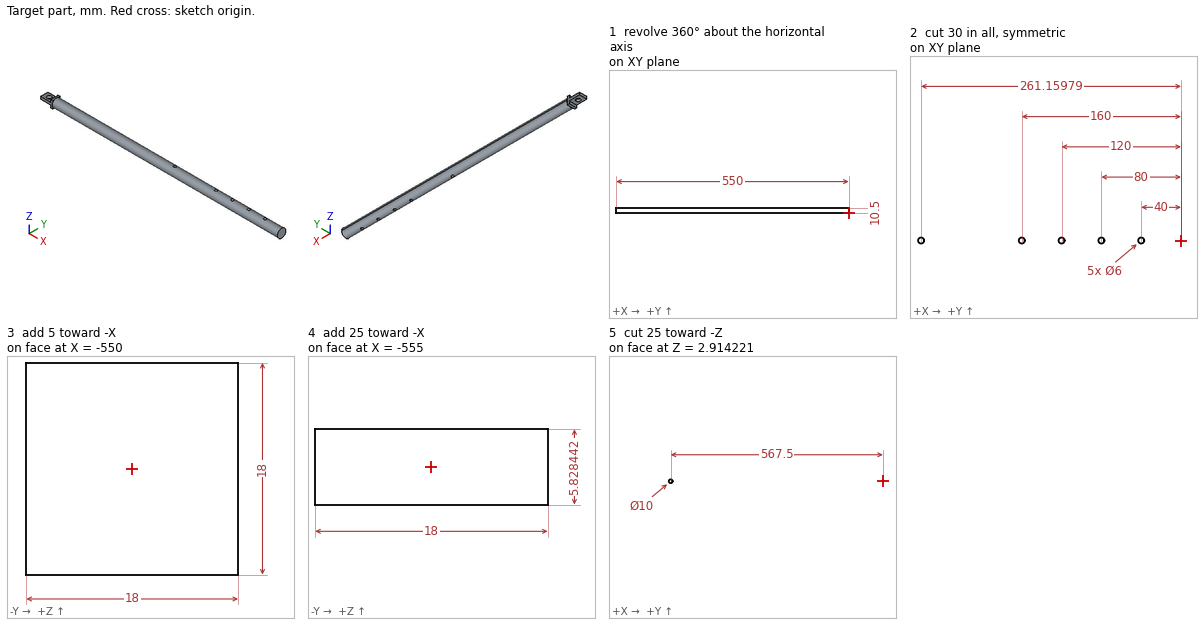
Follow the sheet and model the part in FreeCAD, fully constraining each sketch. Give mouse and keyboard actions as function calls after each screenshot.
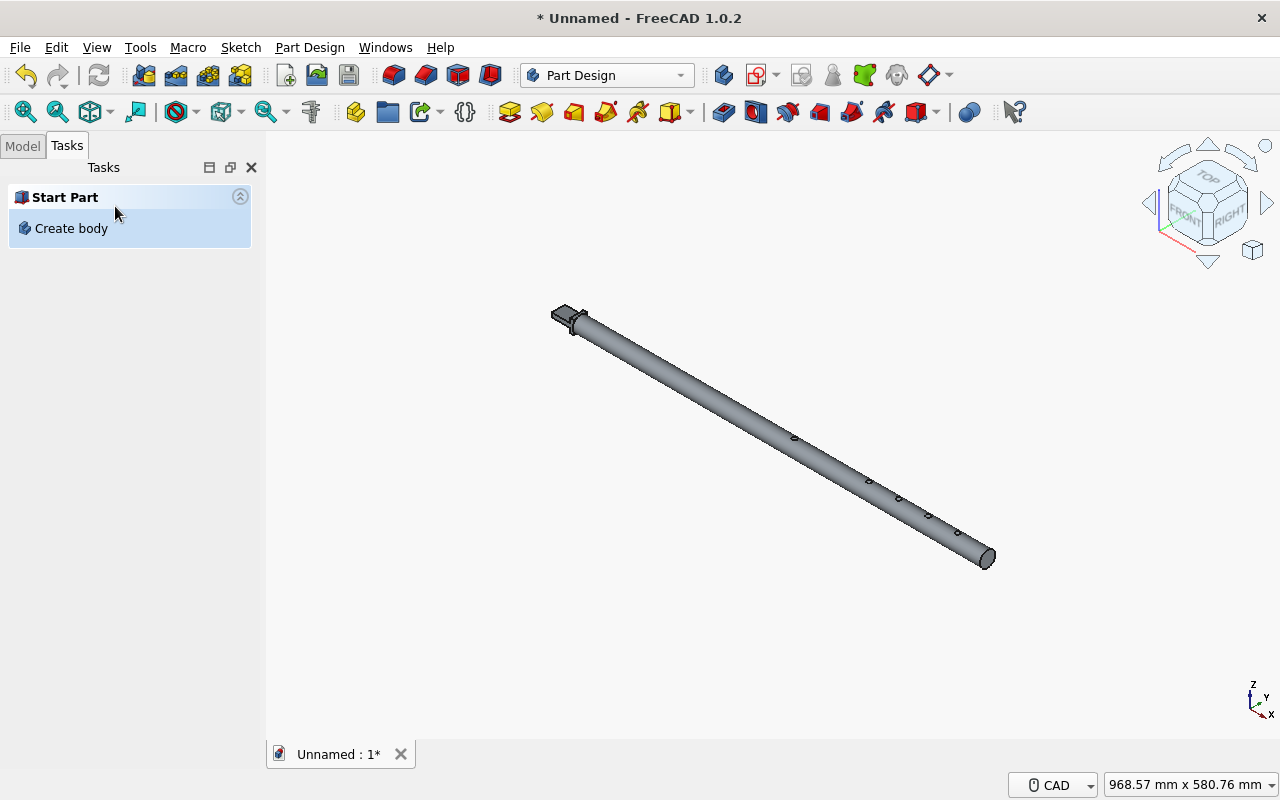
key(2)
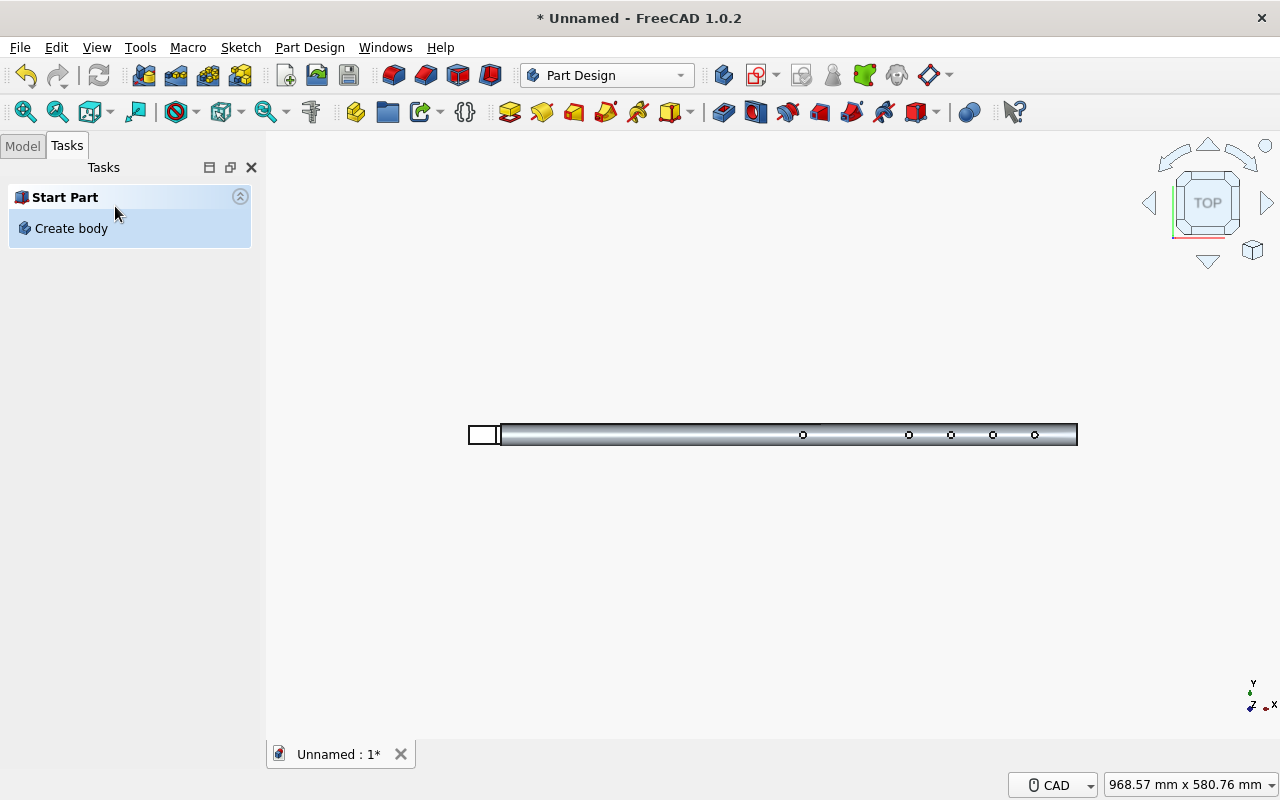
click(482, 434)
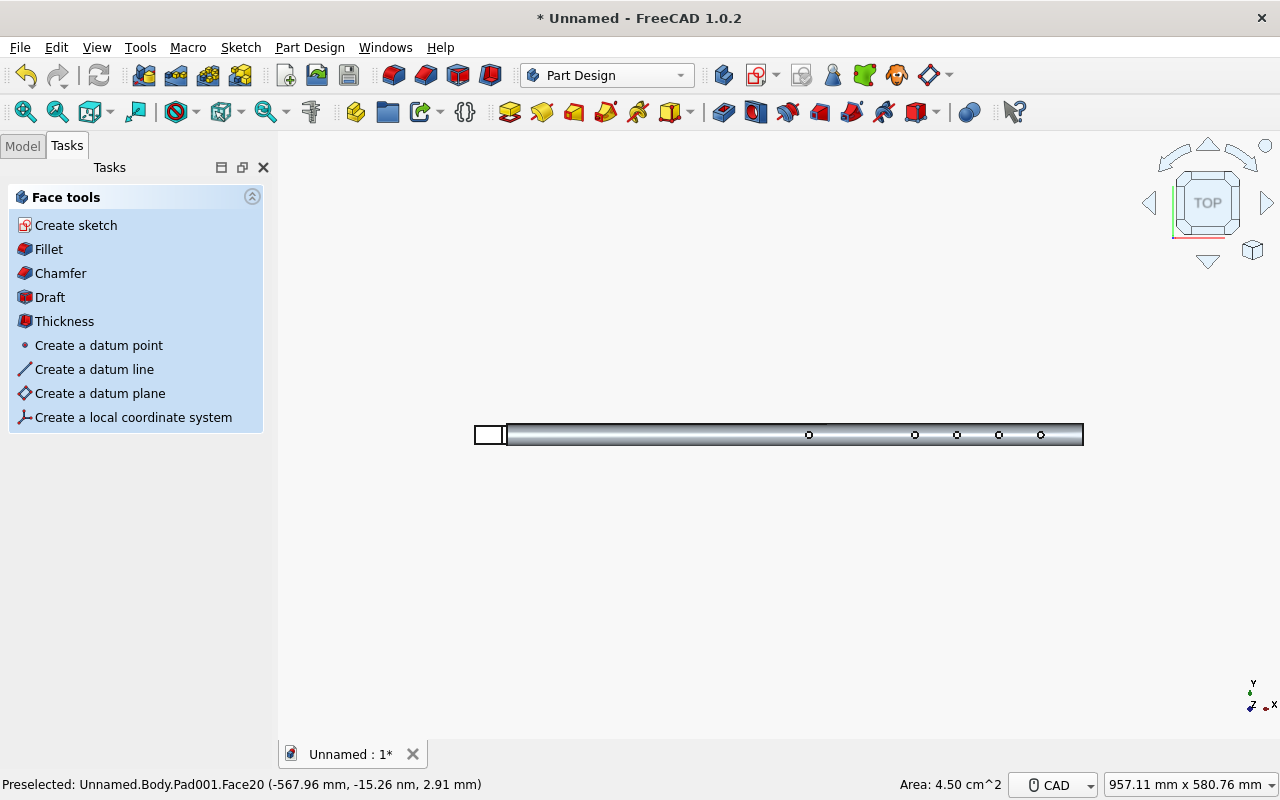
click(756, 76)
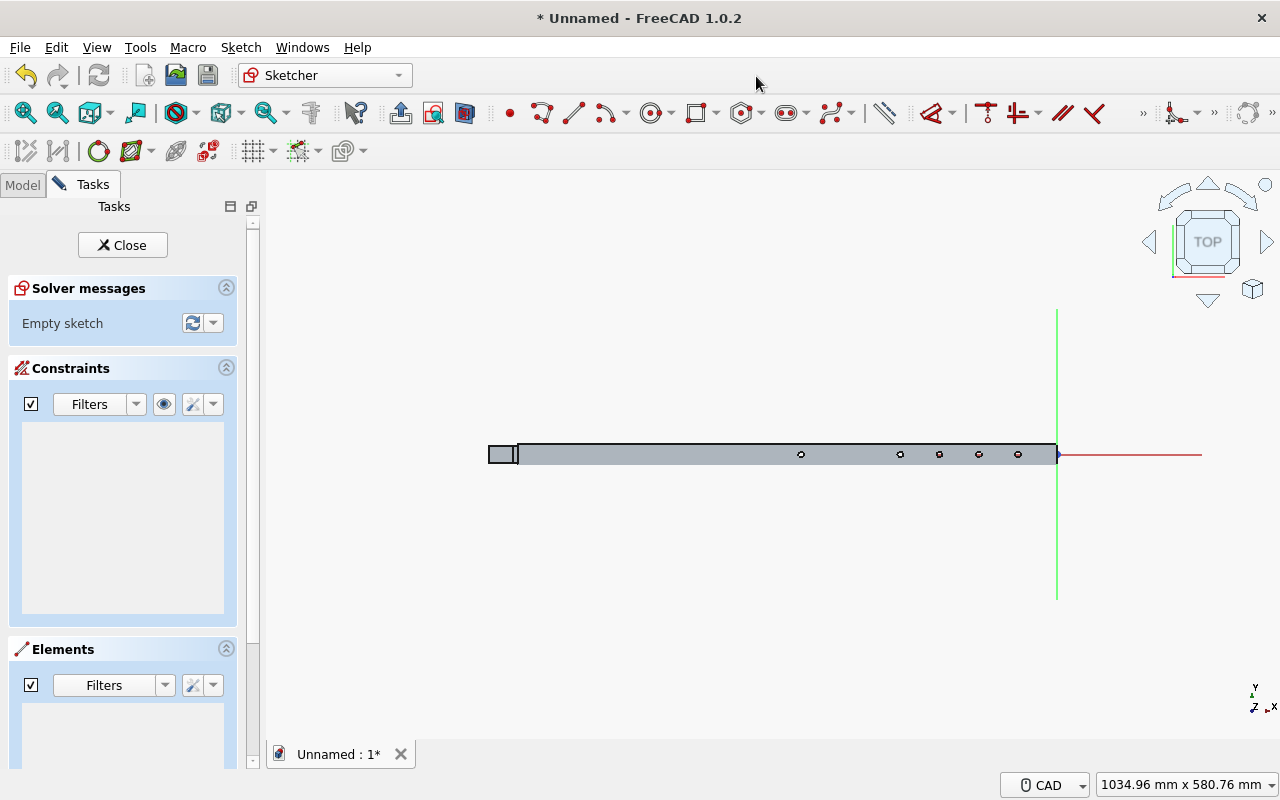
scroll(490, 454, up, 15)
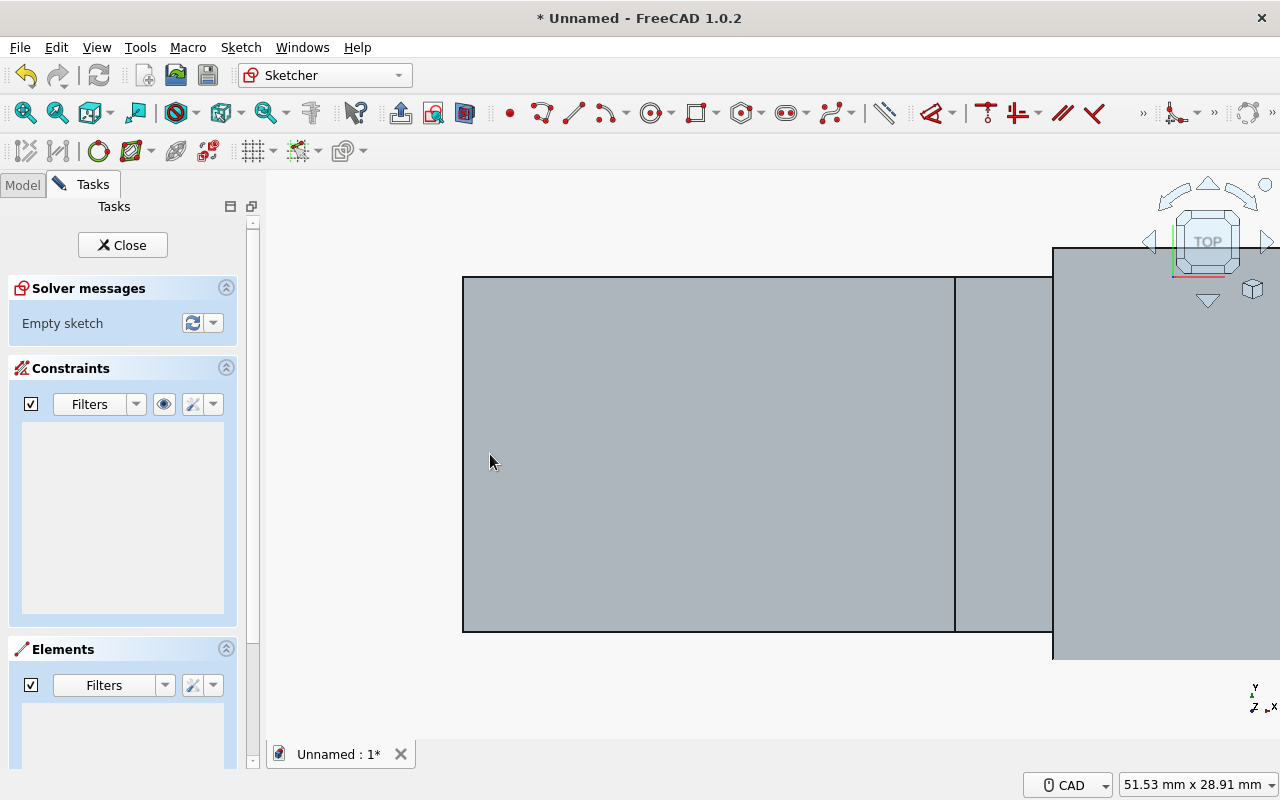
scroll(715, 454, up, 3)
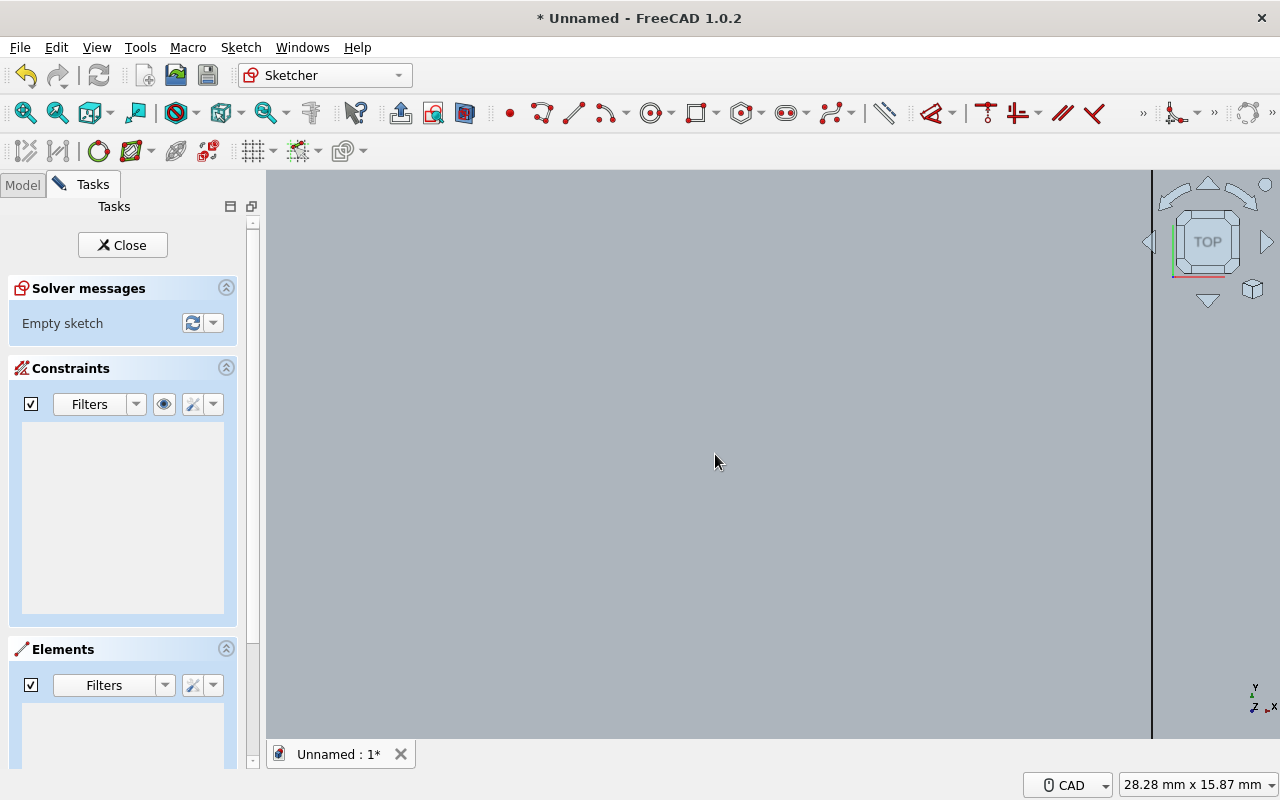
key(g)
key(c)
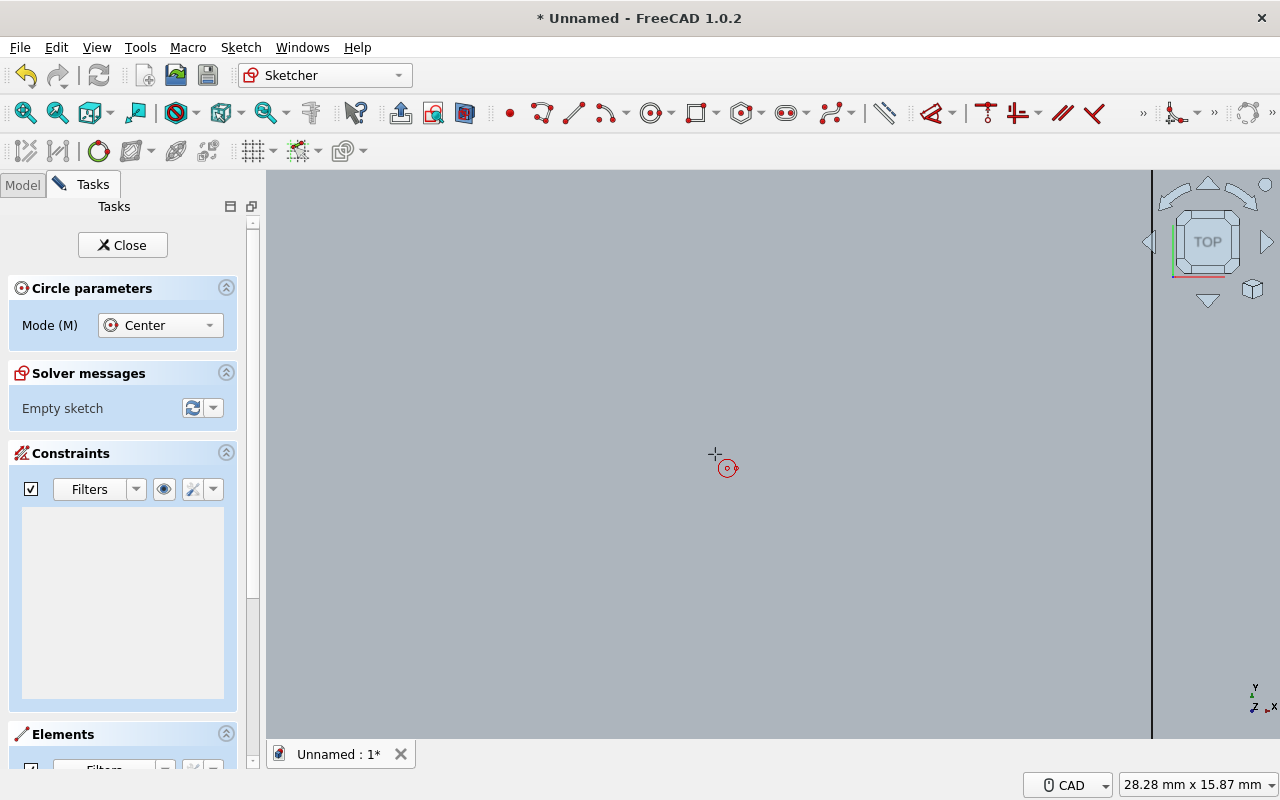
click(704, 454)
click(831, 328)
key(Escape)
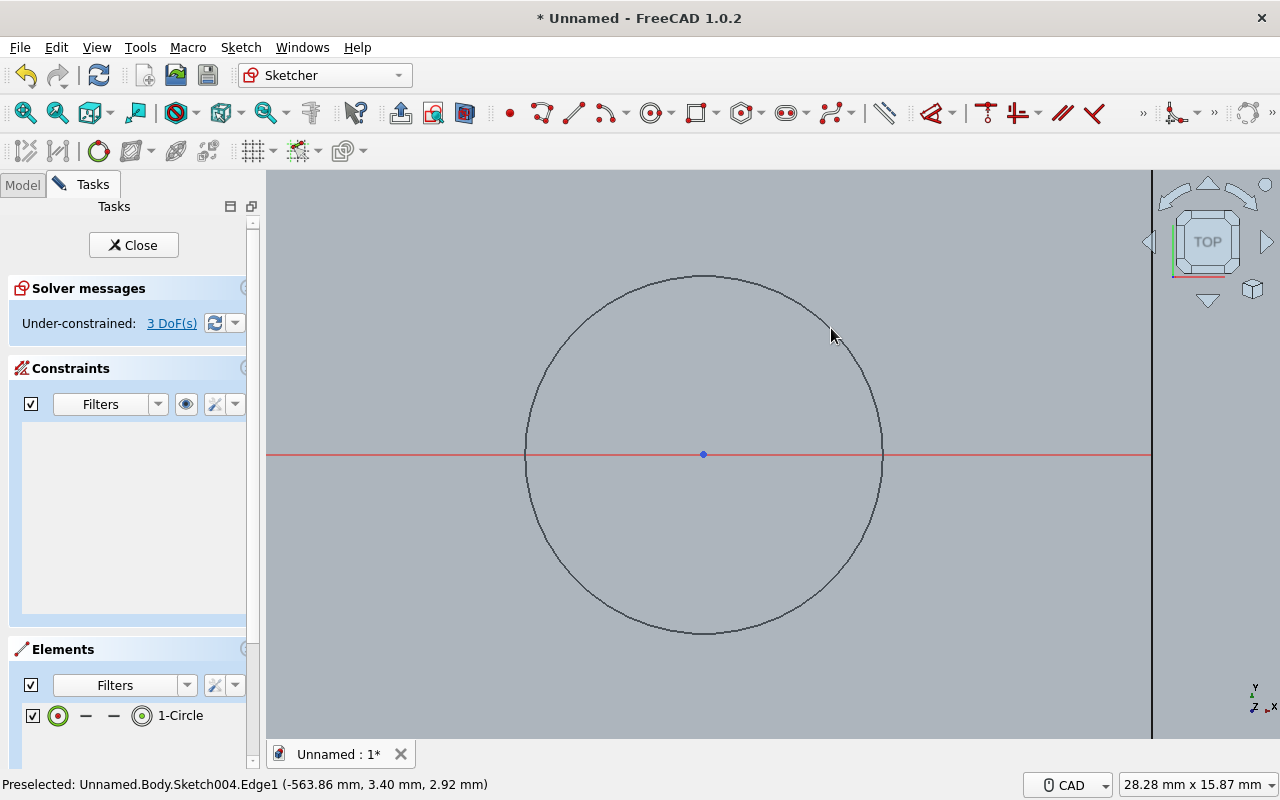
click(704, 455)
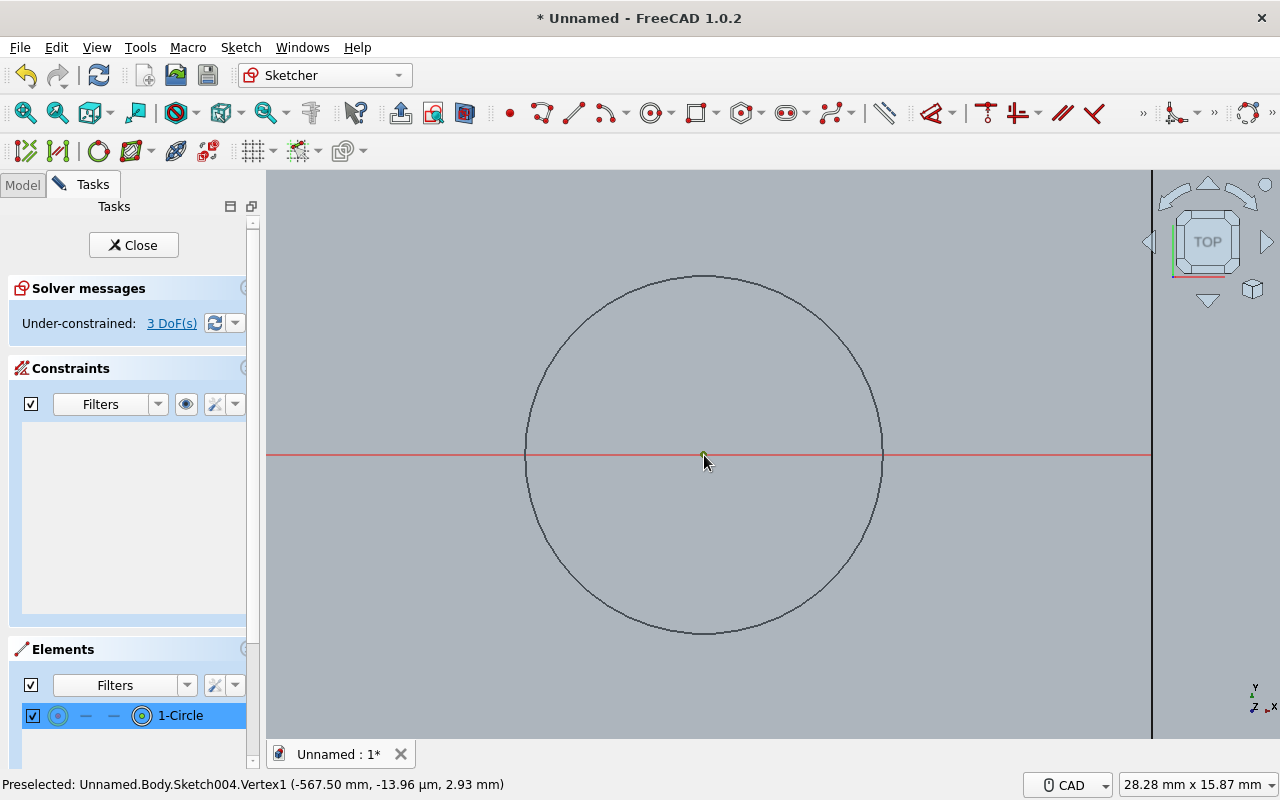
click(353, 454)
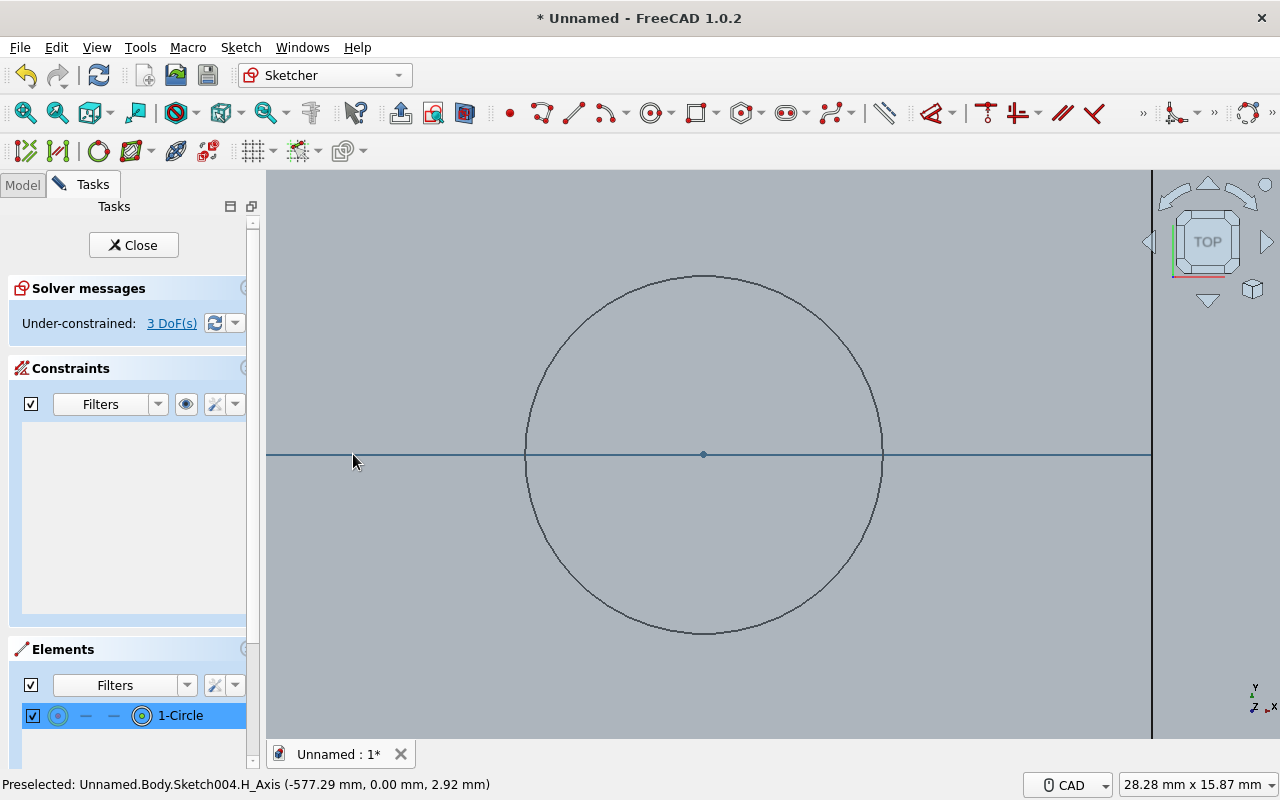
key(c)